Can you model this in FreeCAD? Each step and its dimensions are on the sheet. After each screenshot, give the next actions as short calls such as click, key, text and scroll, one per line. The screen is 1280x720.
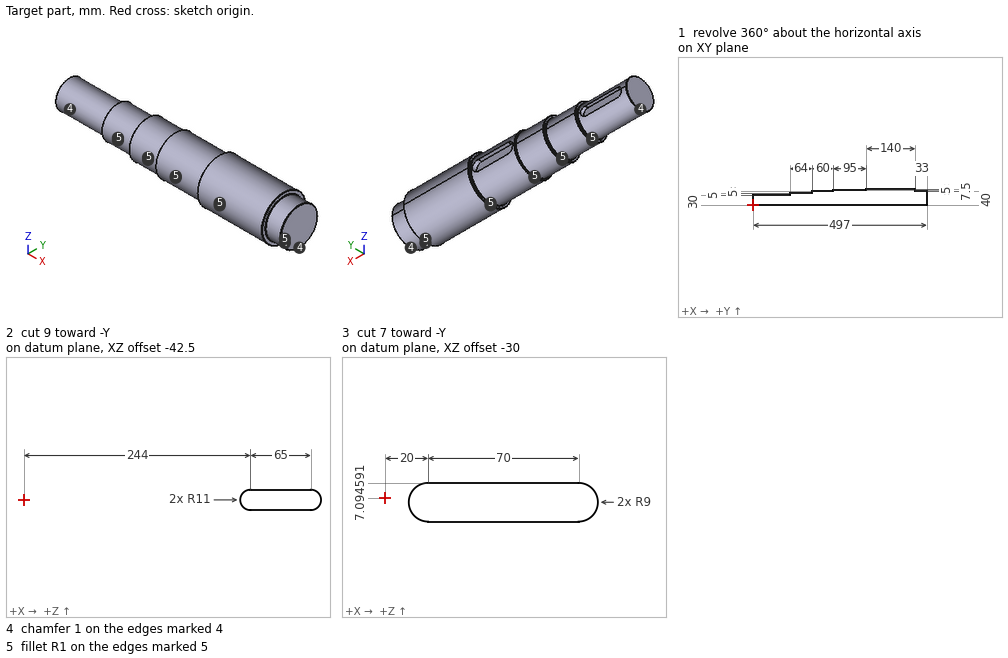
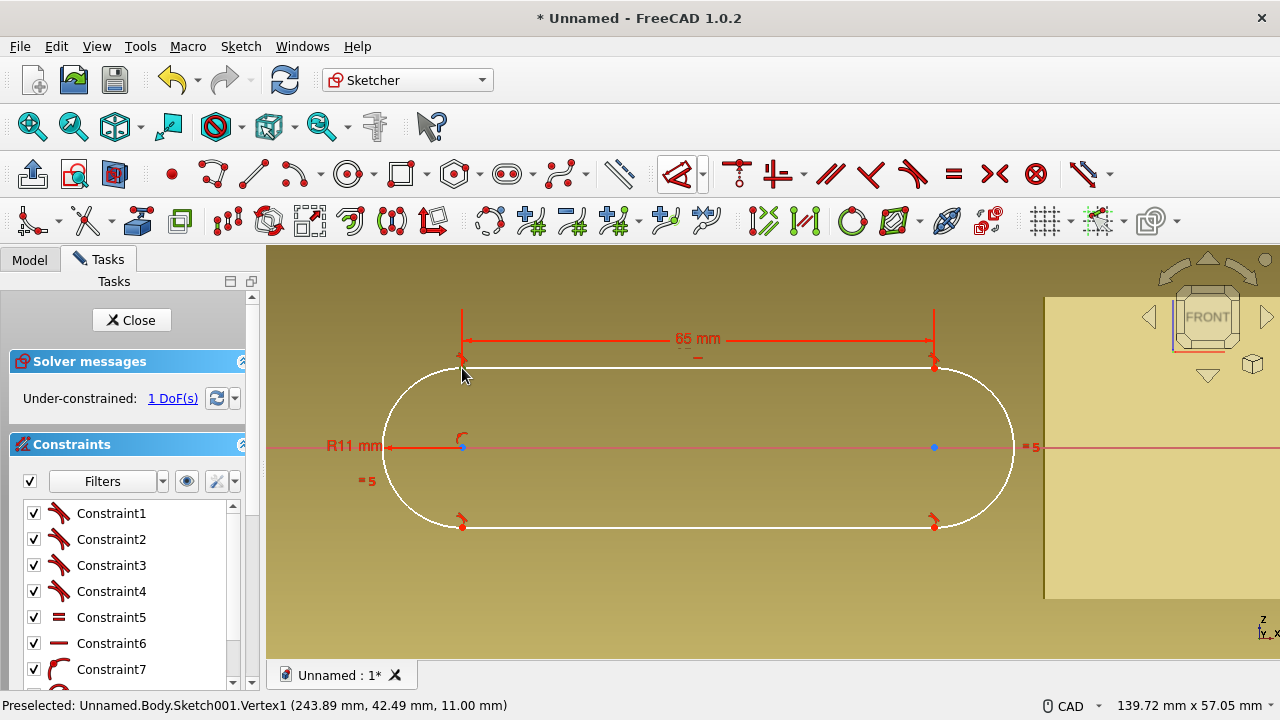
key(l)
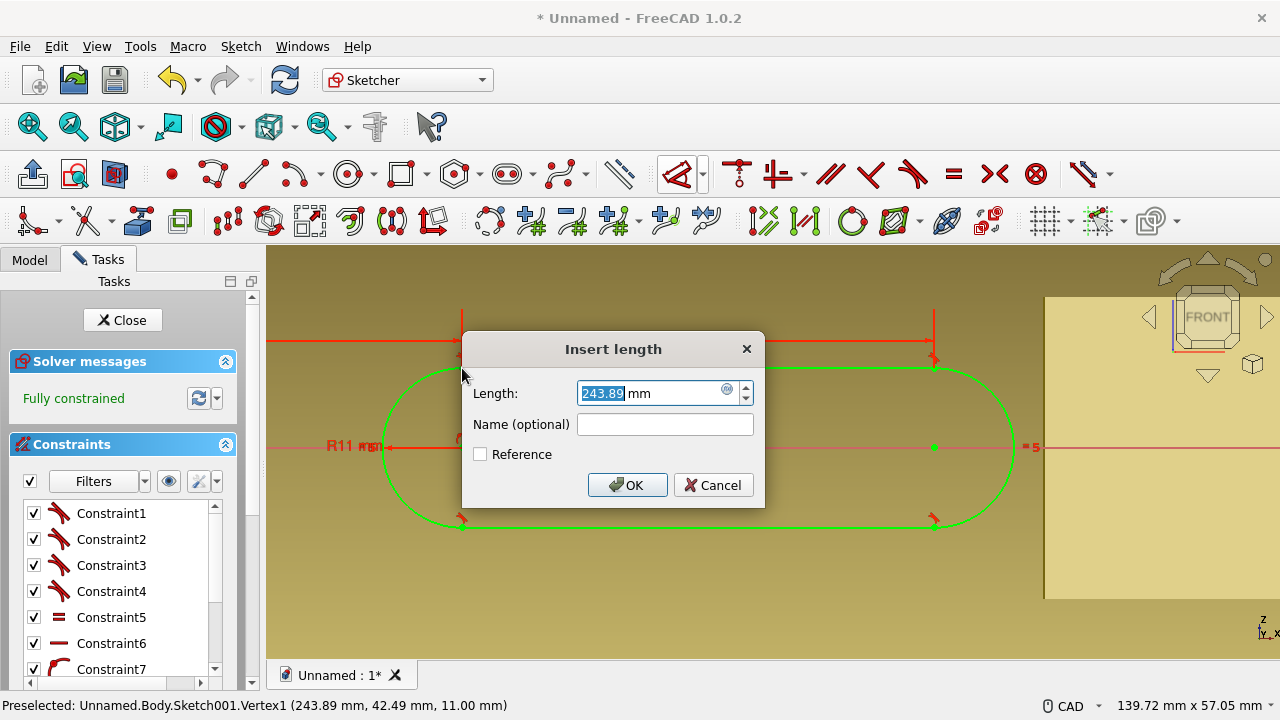
text(244)
key(Return)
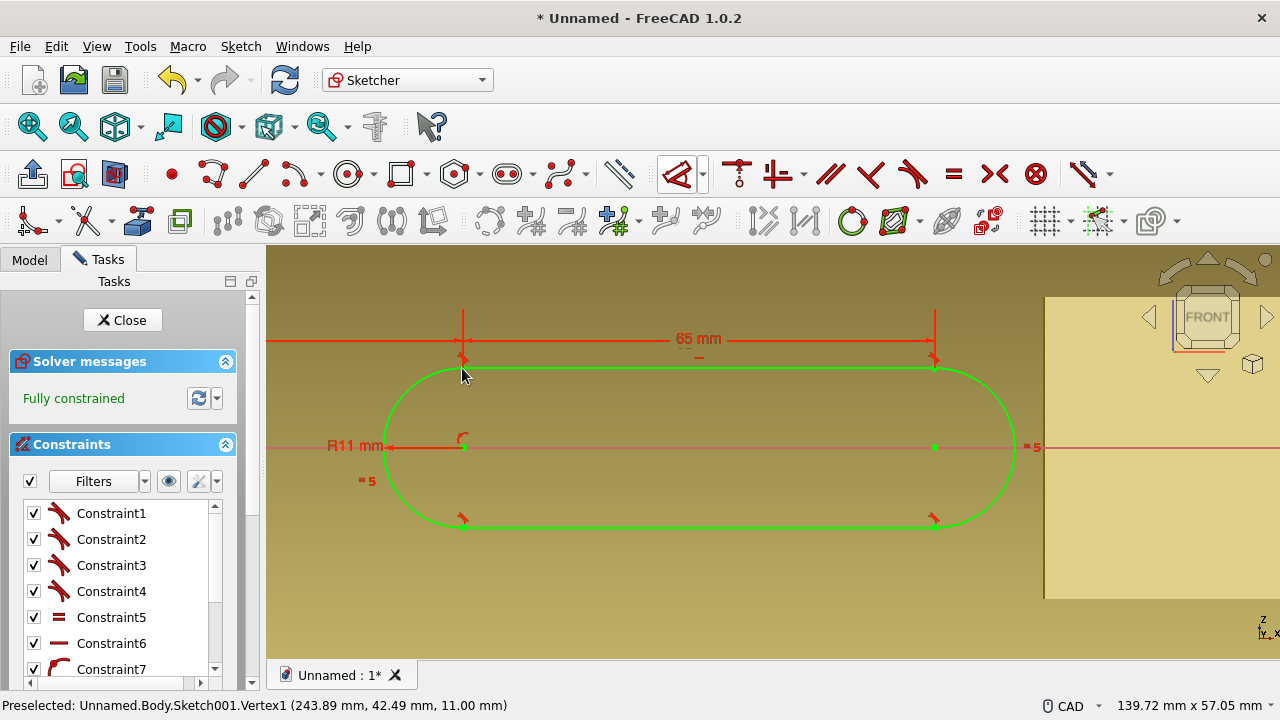
click(123, 320)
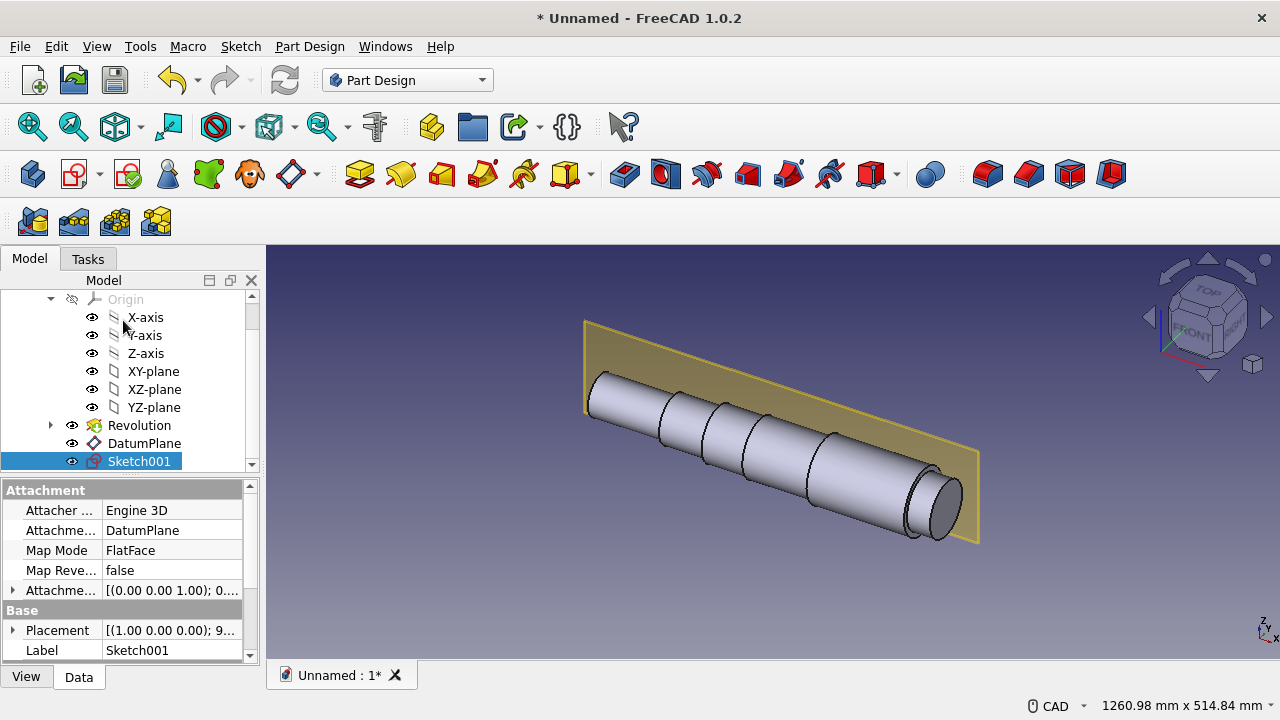
click(625, 174)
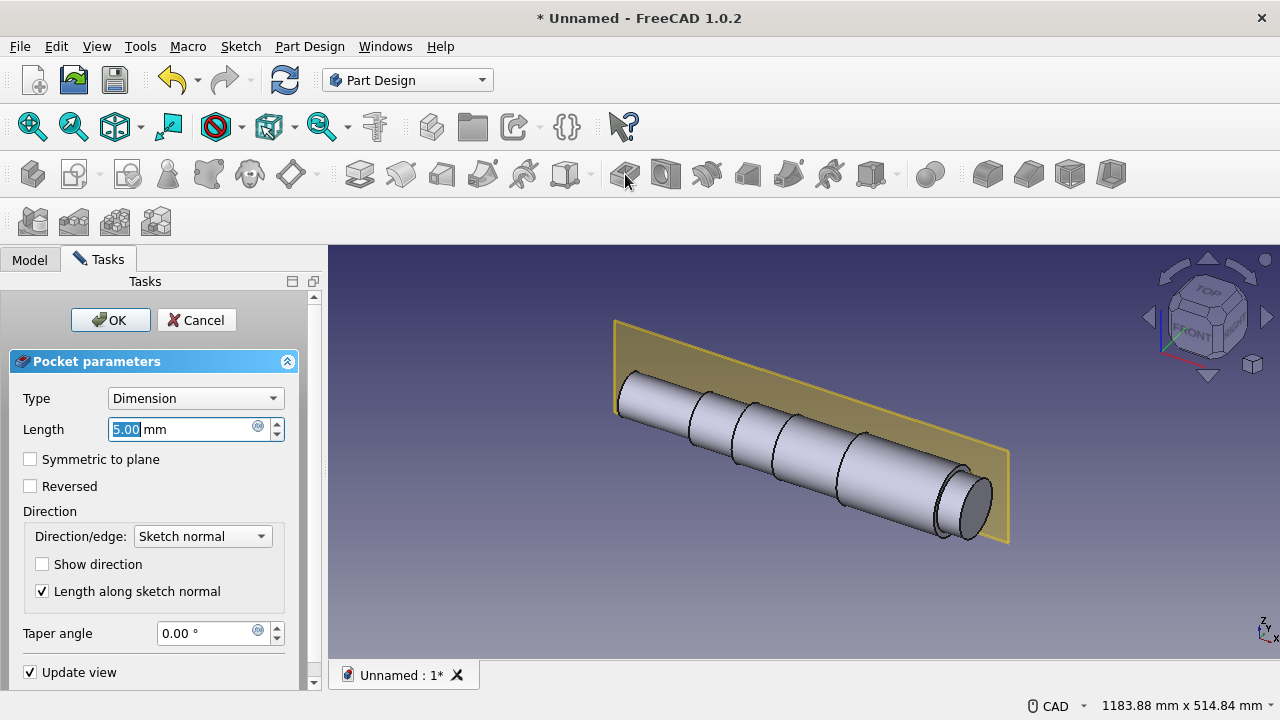
text(9)
key(Tab)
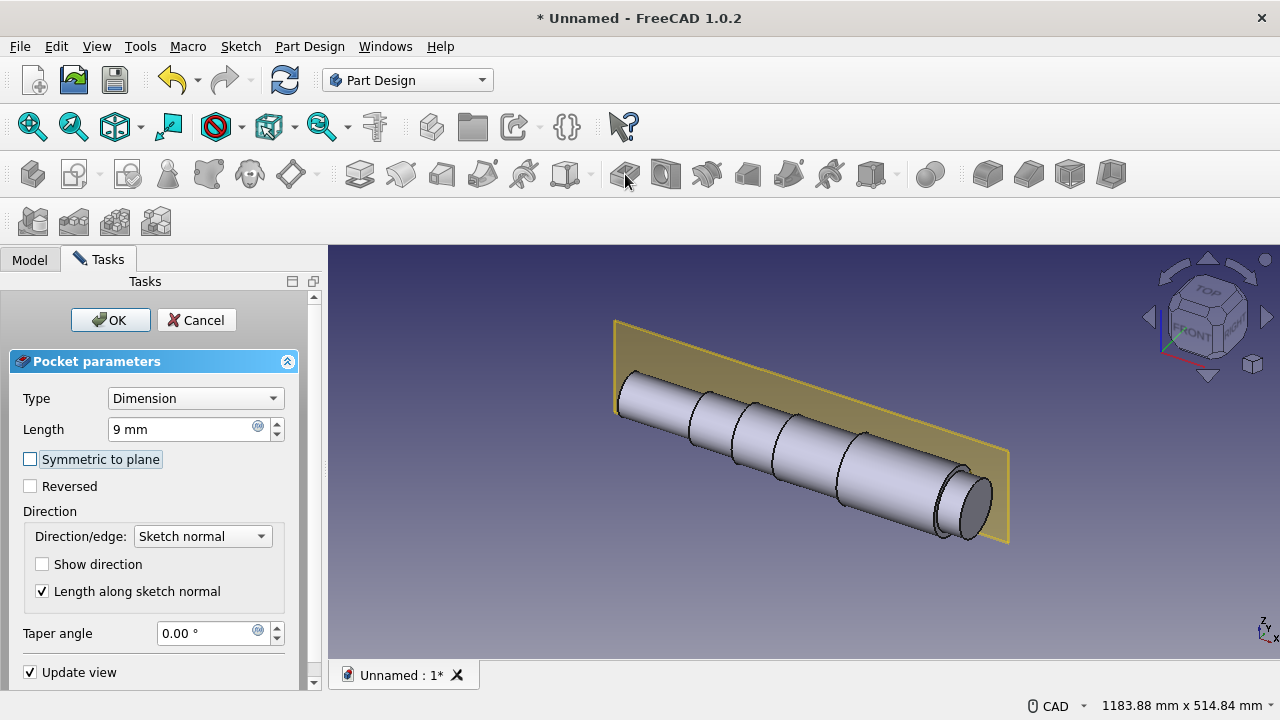
click(31, 486)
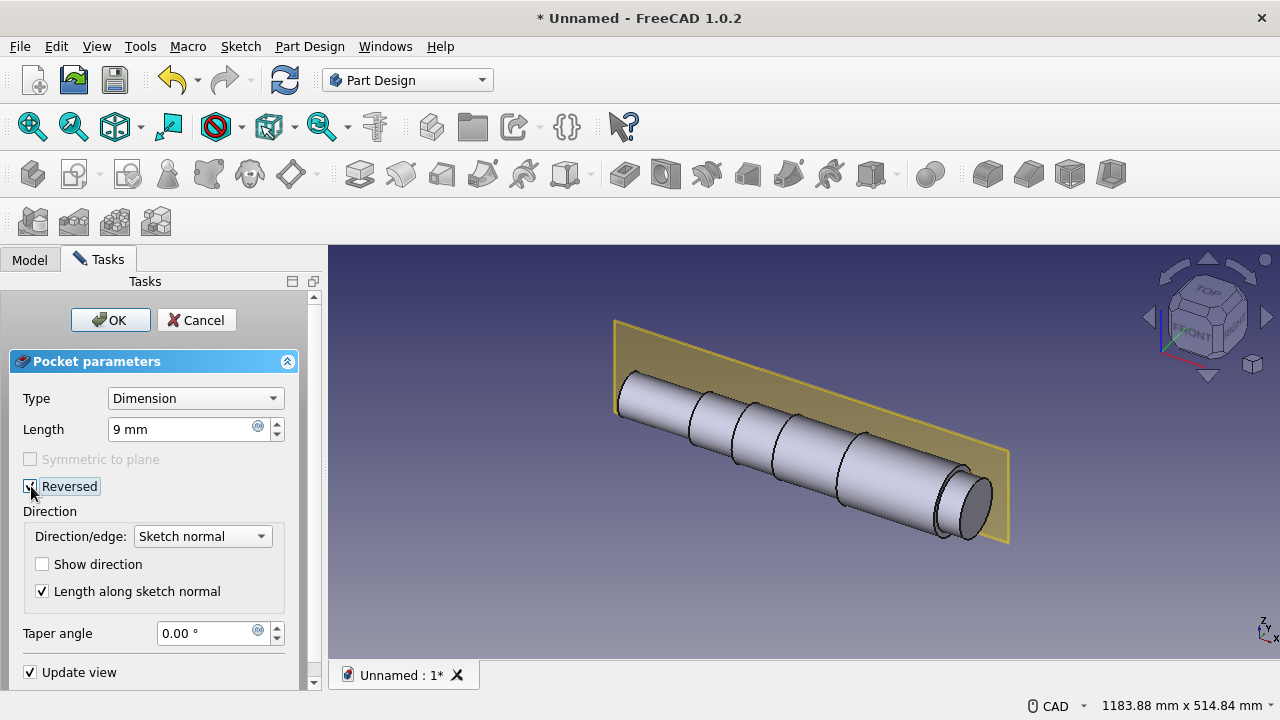
click(111, 320)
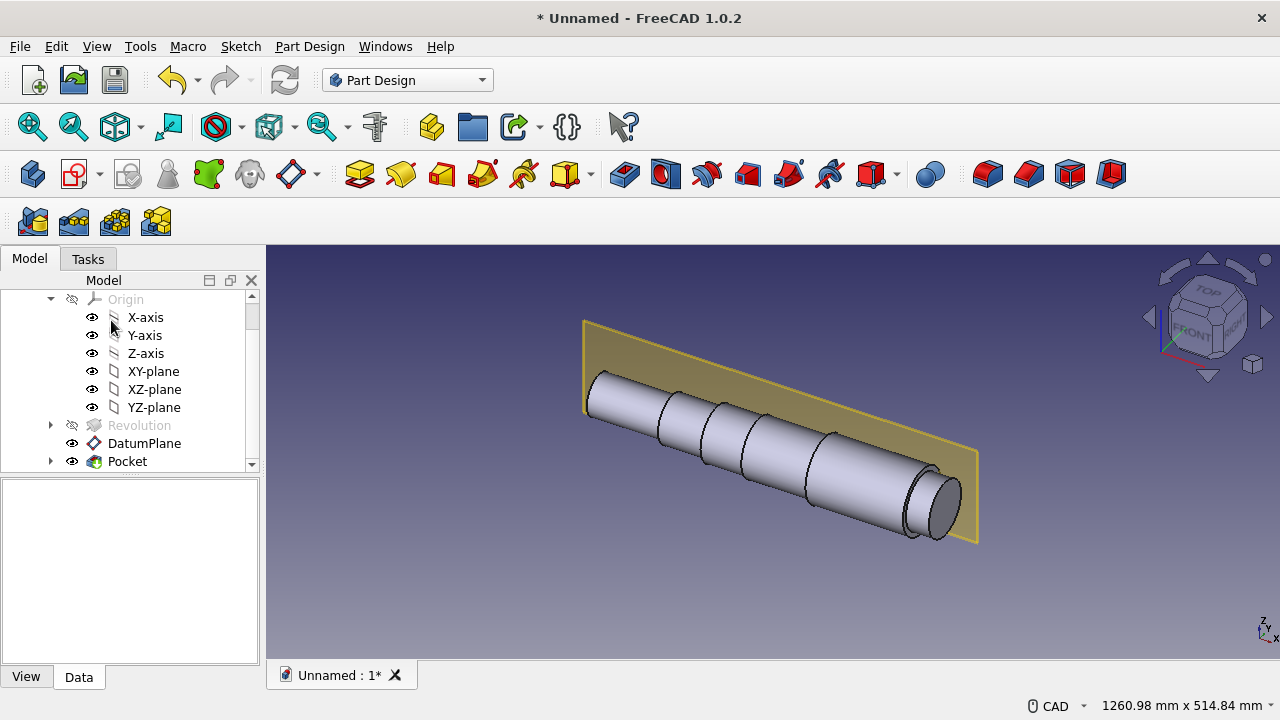
click(117, 443)
key(space)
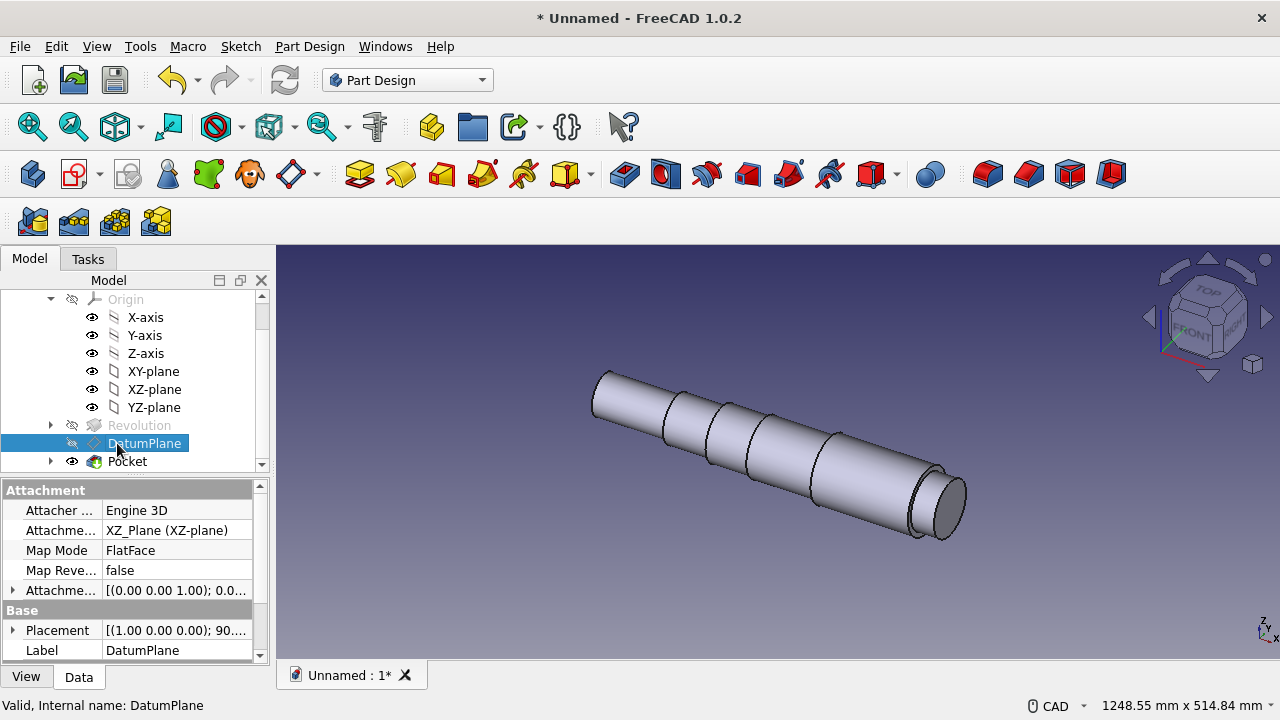
click(137, 389)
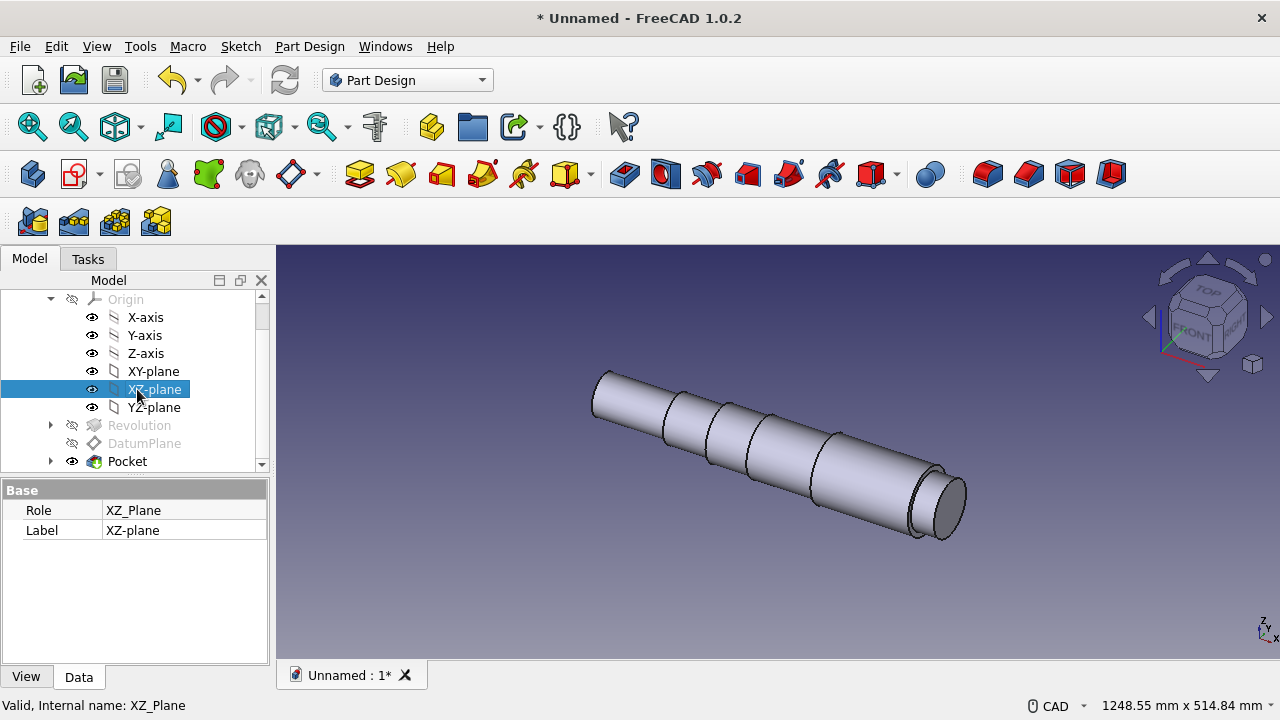
click(290, 174)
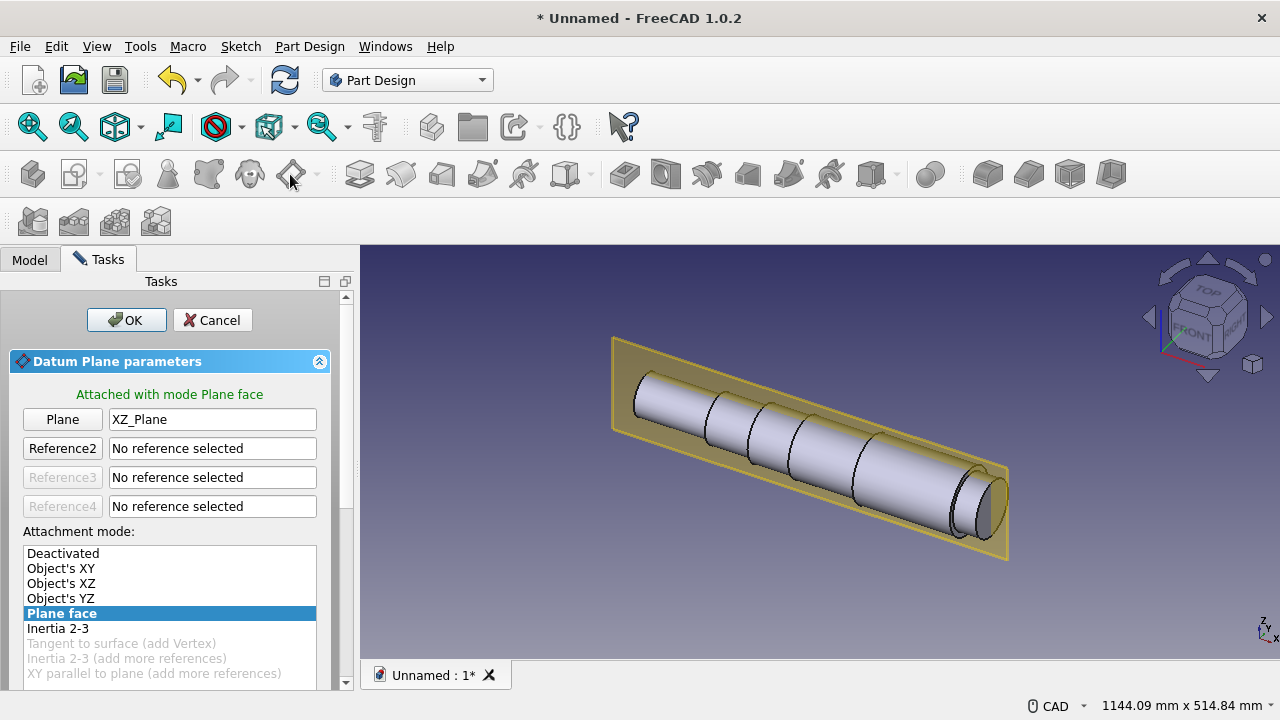
scroll(346, 490, down, 4)